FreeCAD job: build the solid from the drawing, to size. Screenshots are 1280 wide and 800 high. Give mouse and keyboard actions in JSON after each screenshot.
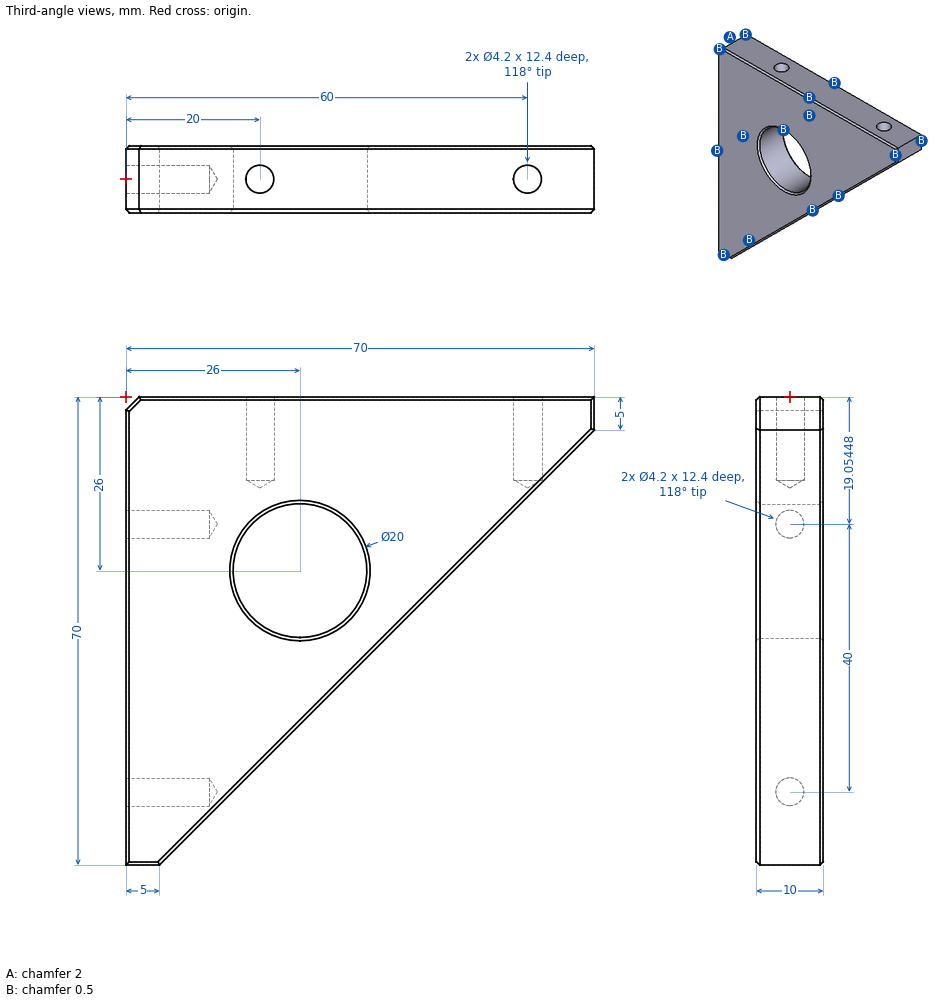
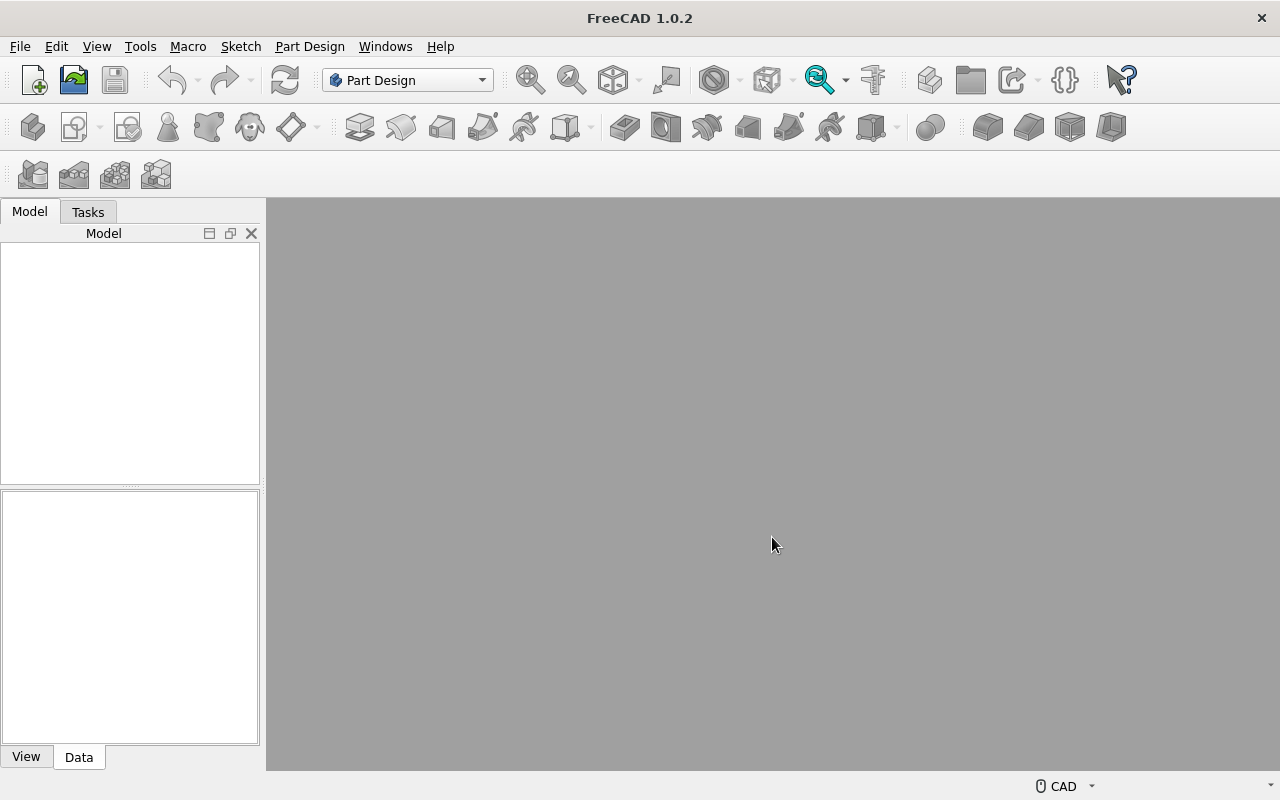
{"action": "left_click", "coordinate": [33, 80]}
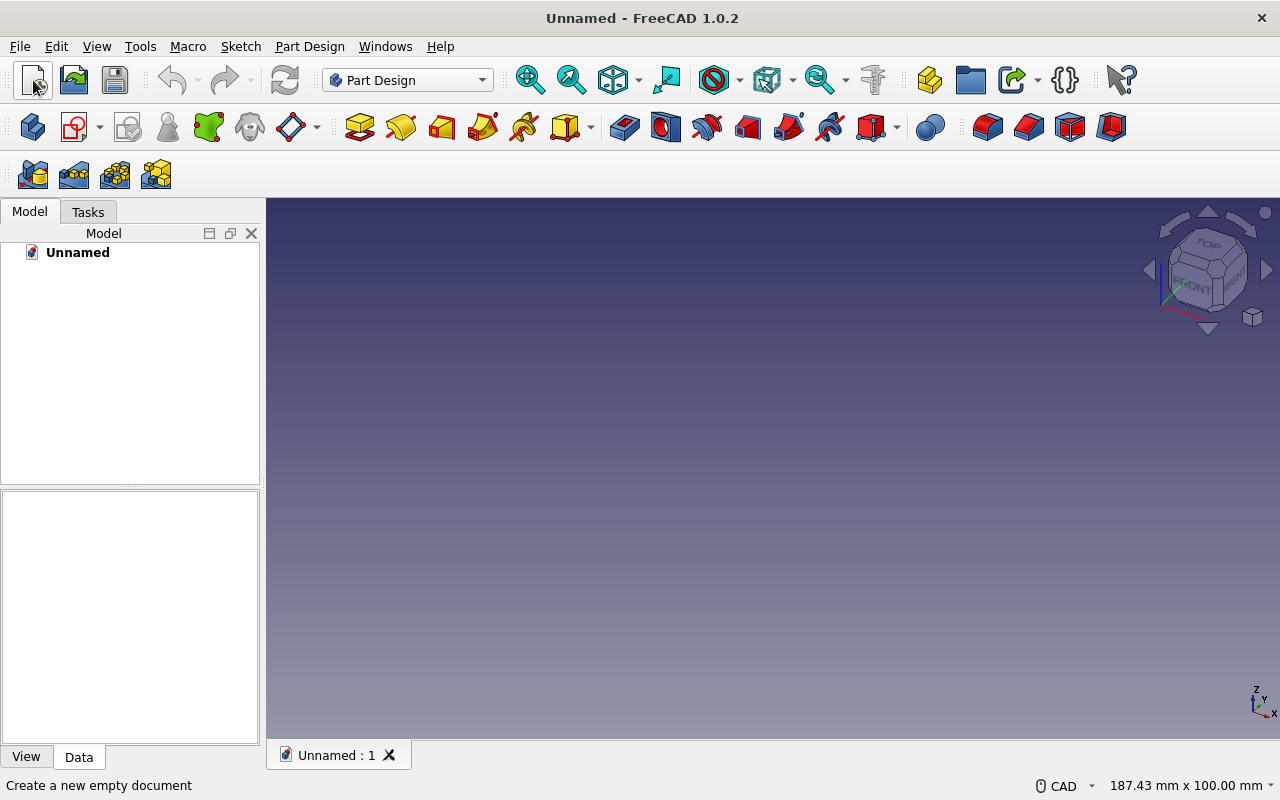
{"action": "left_click", "coordinate": [74, 128]}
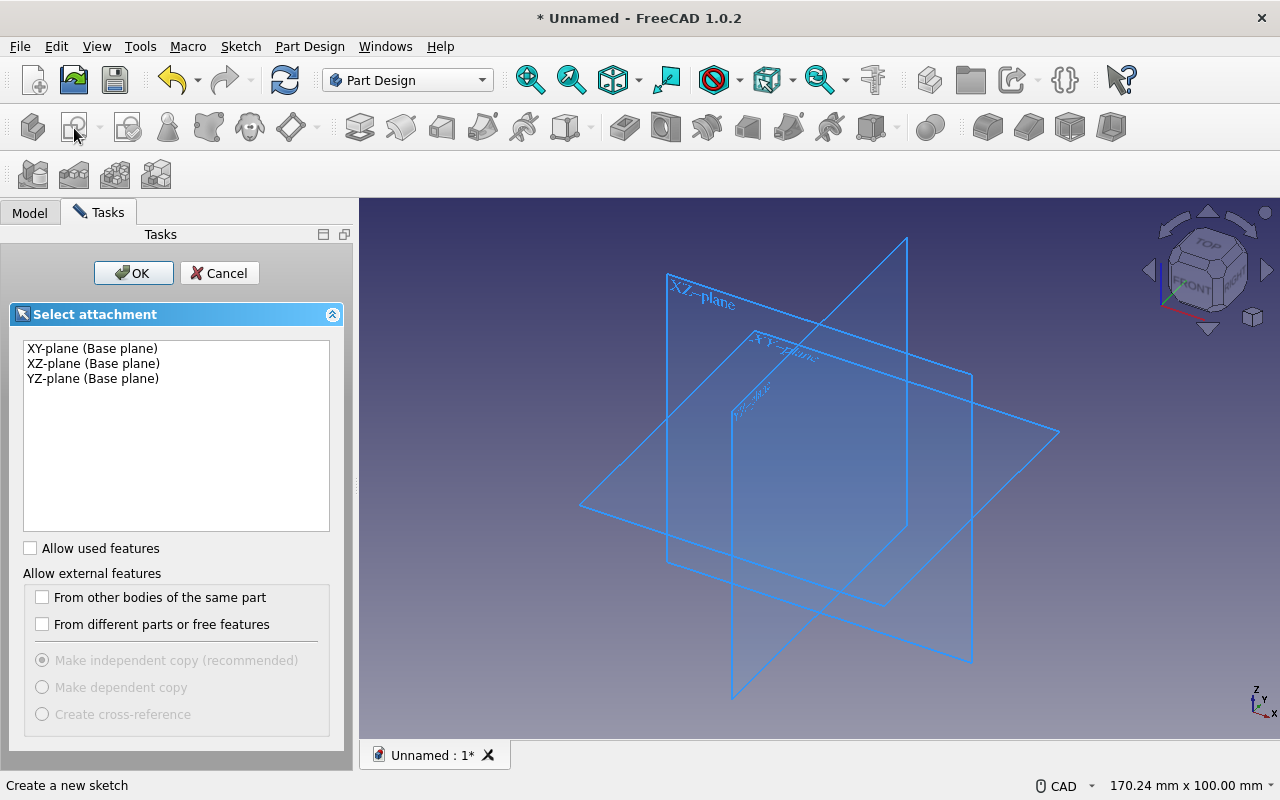
{"action": "left_click", "coordinate": [84, 364]}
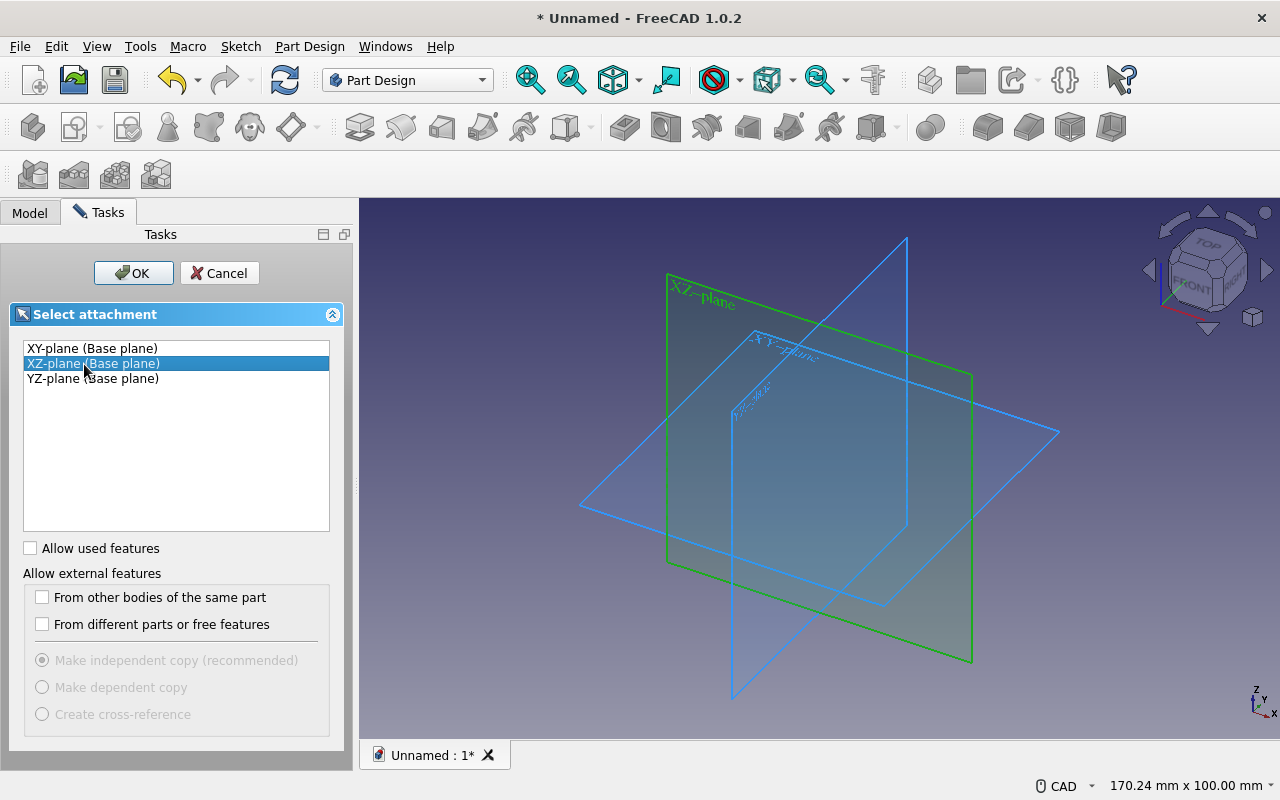
{"action": "left_click", "coordinate": [134, 273]}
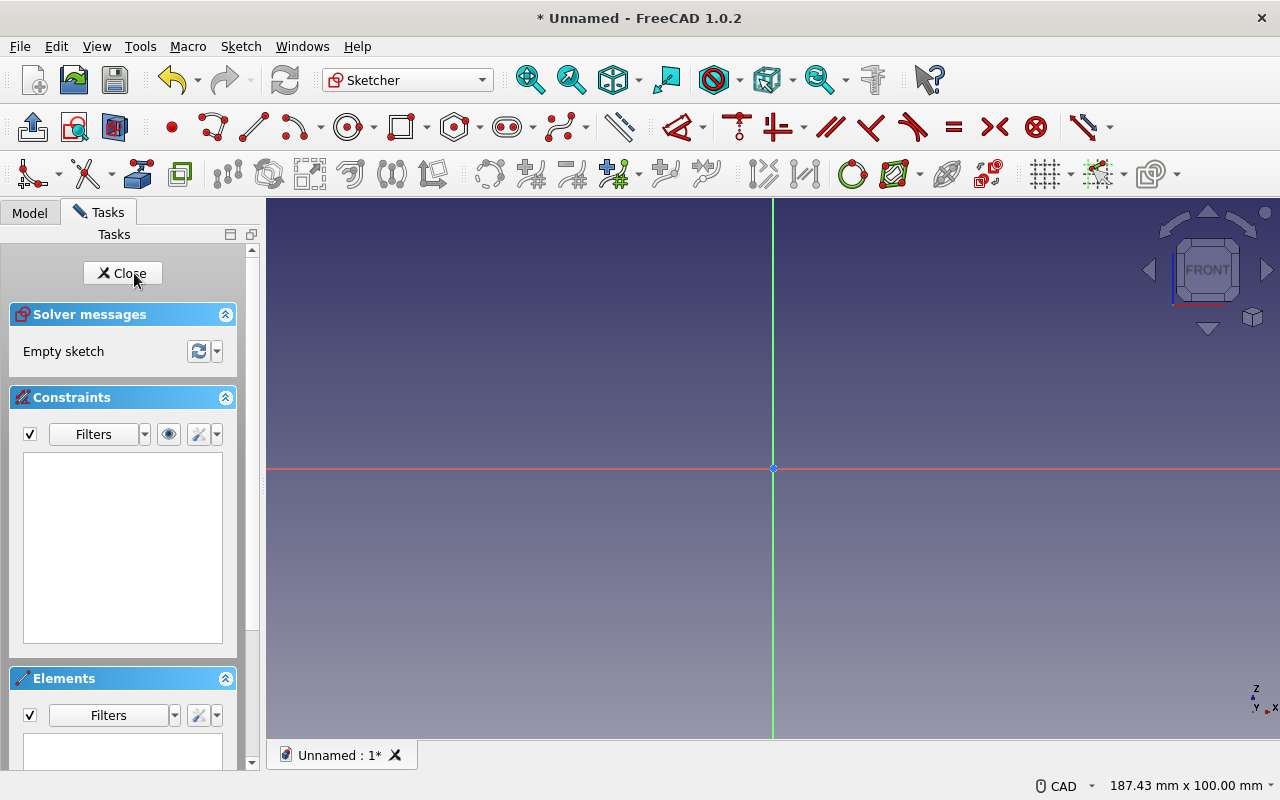
{"action": "scroll", "coordinate": [294, 226], "scroll_direction": "down", "scroll_amount": 2}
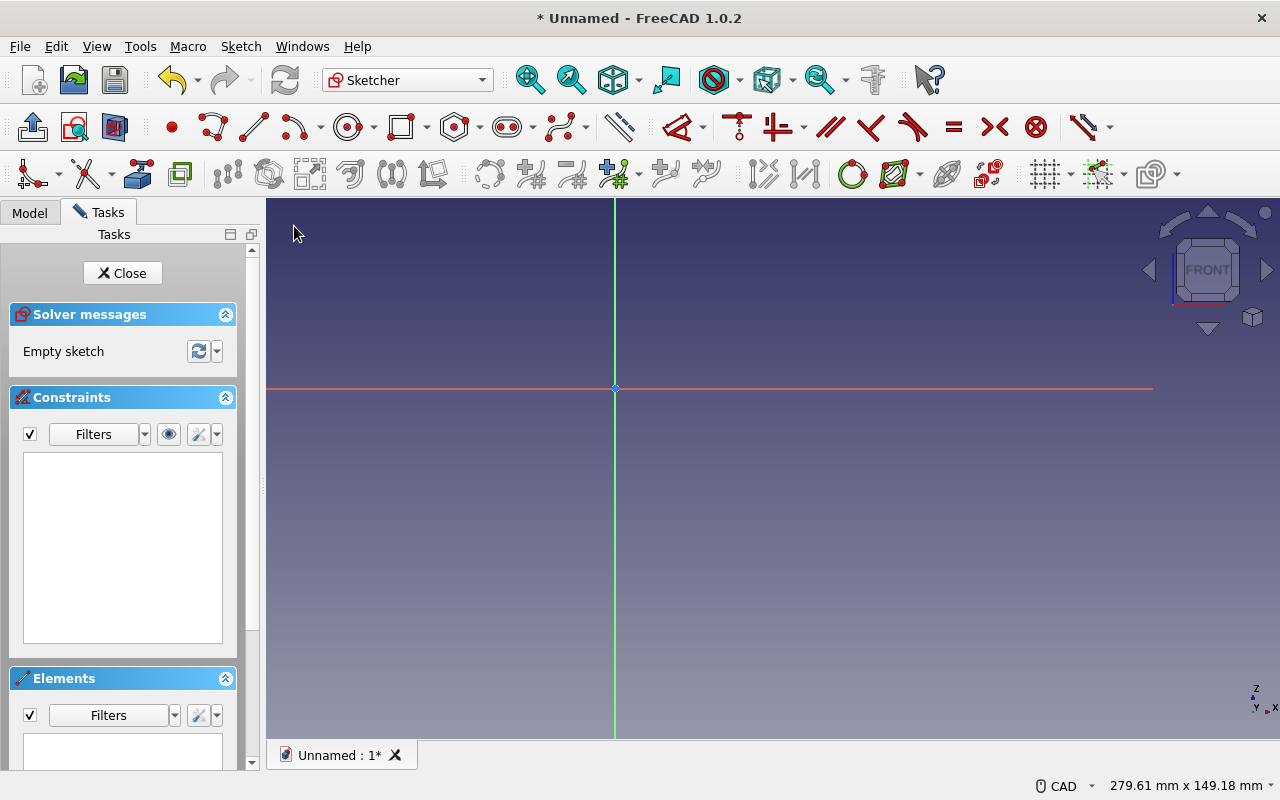
{"action": "left_click", "coordinate": [213, 128]}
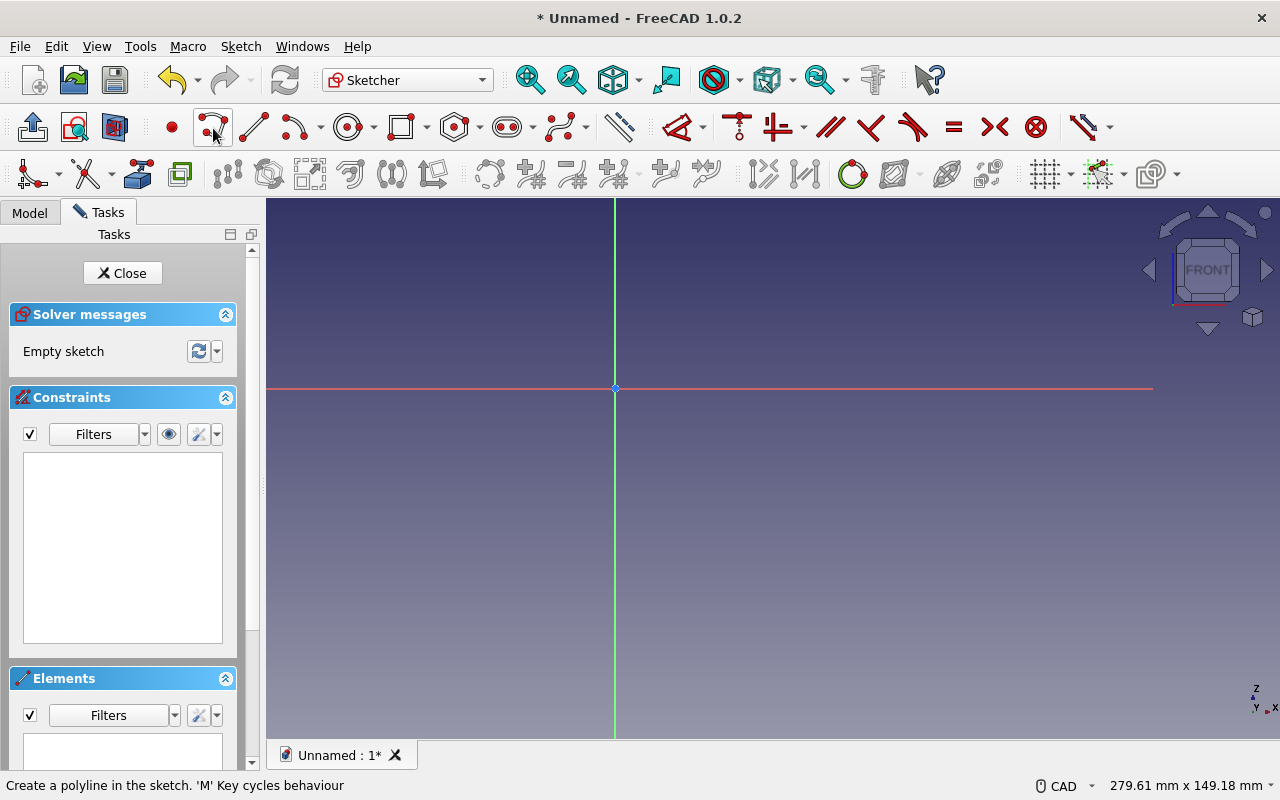
{"action": "left_click", "coordinate": [615, 389]}
{"action": "left_click", "coordinate": [869, 398]}
{"action": "left_click", "coordinate": [869, 407]}
{"action": "left_click", "coordinate": [633, 642]}
{"action": "left_click", "coordinate": [624, 642]}
{"action": "left_click", "coordinate": [615, 389]}
{"action": "key", "text": "Escape"}
{"action": "key", "text": "Escape"}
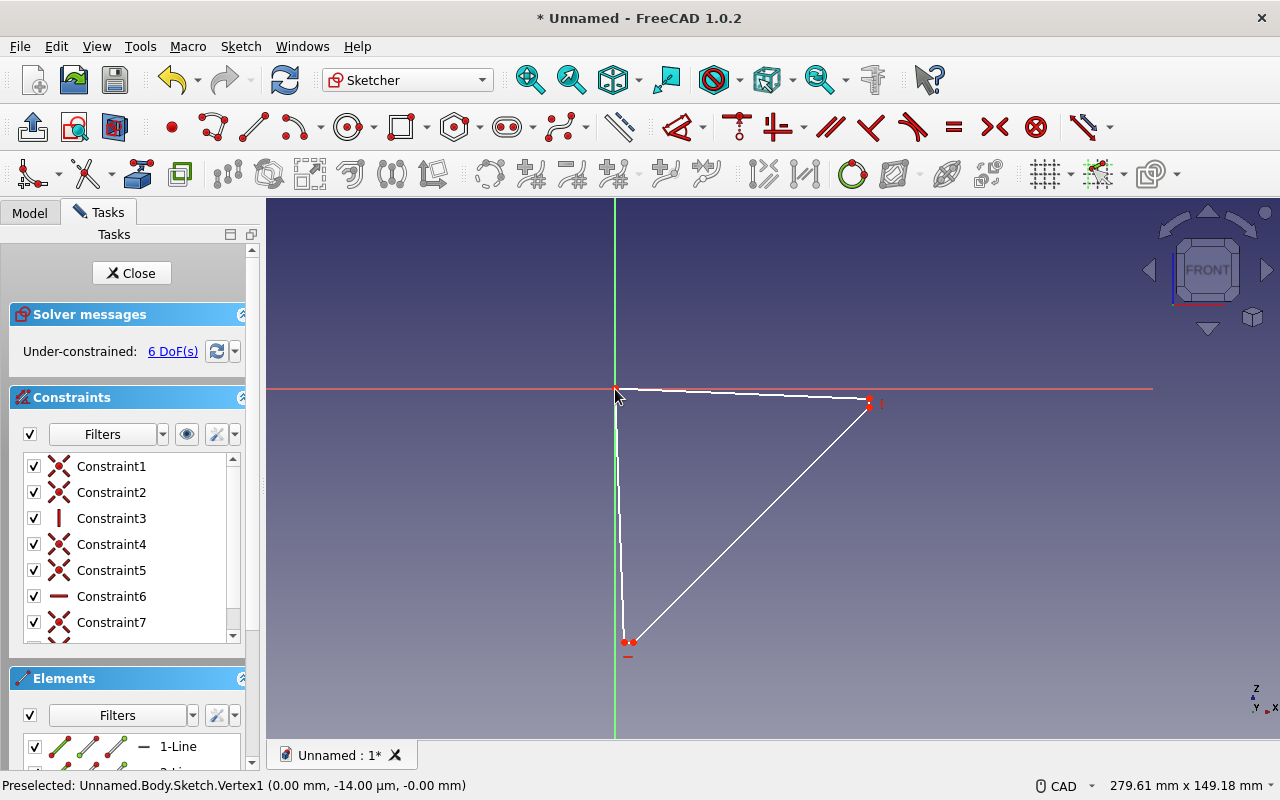
{"action": "left_click", "coordinate": [691, 392]}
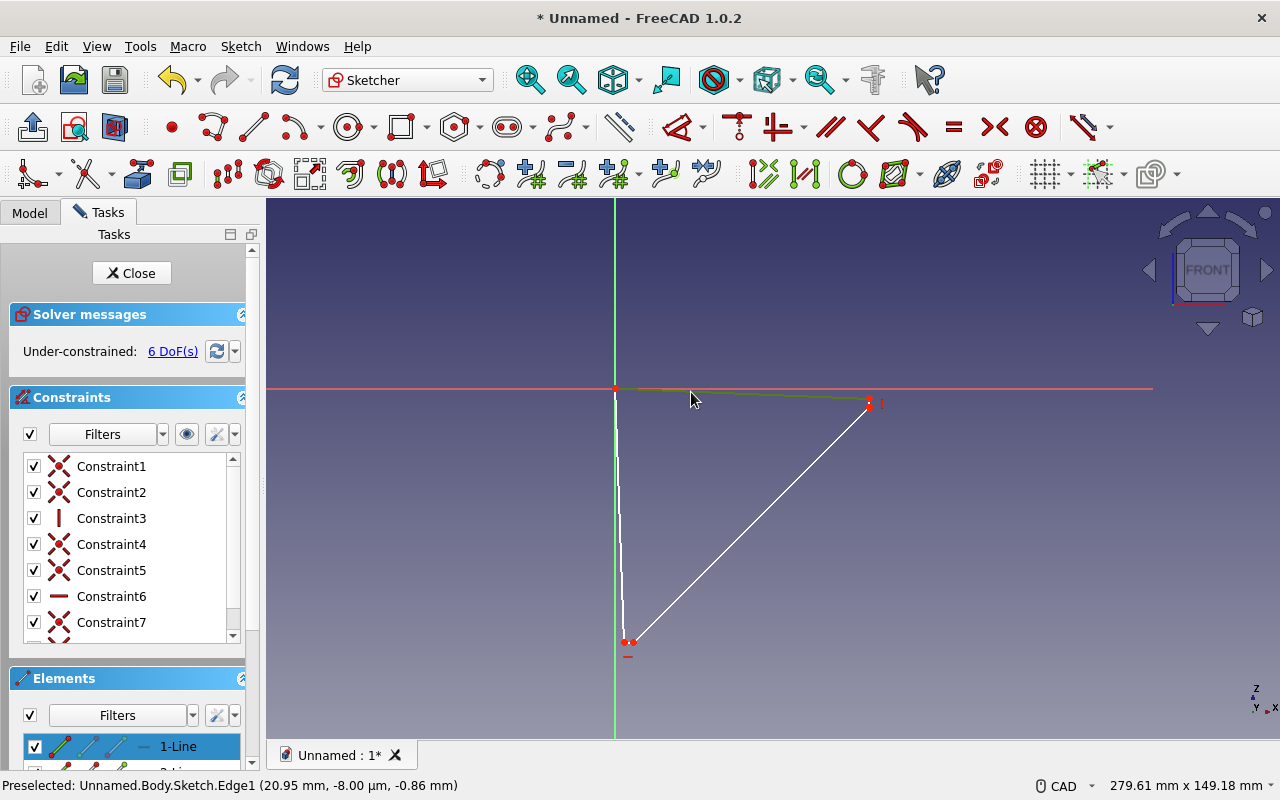
{"action": "left_click", "coordinate": [804, 128]}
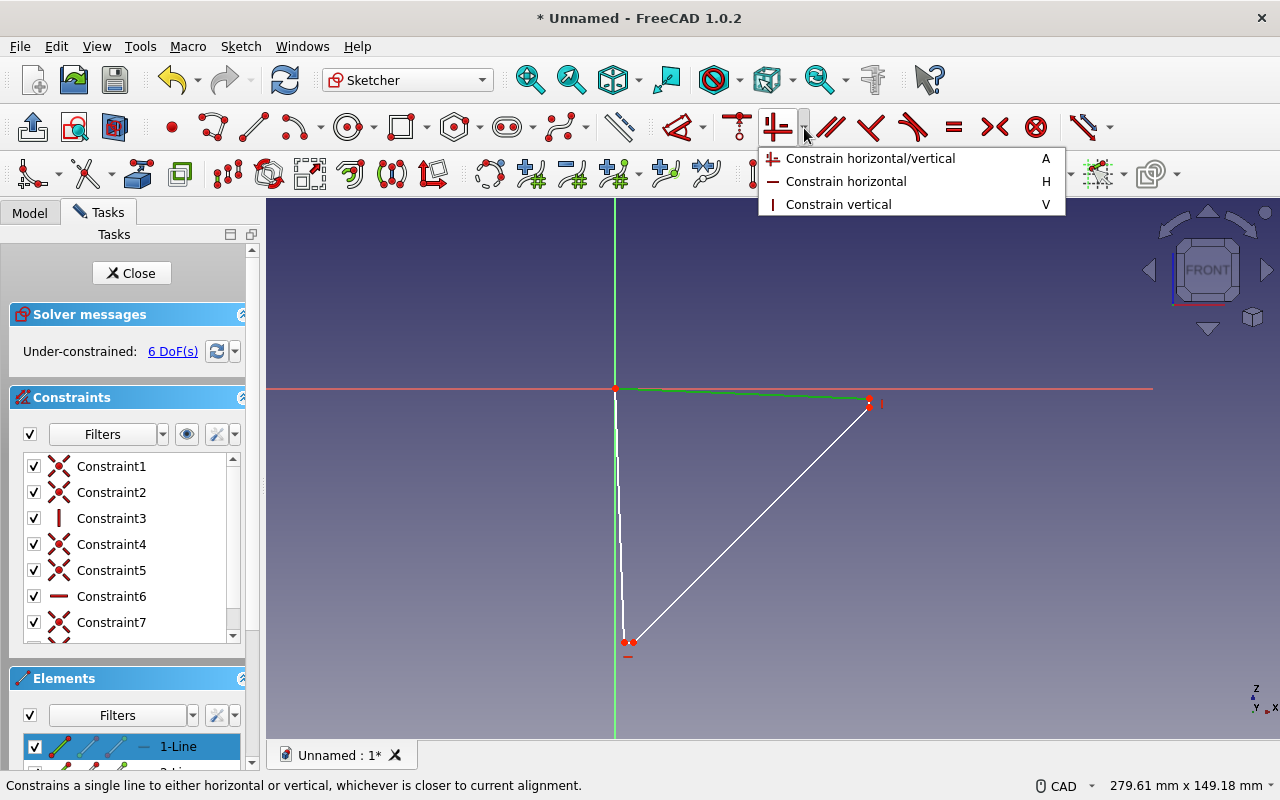
{"action": "left_click", "coordinate": [912, 182]}